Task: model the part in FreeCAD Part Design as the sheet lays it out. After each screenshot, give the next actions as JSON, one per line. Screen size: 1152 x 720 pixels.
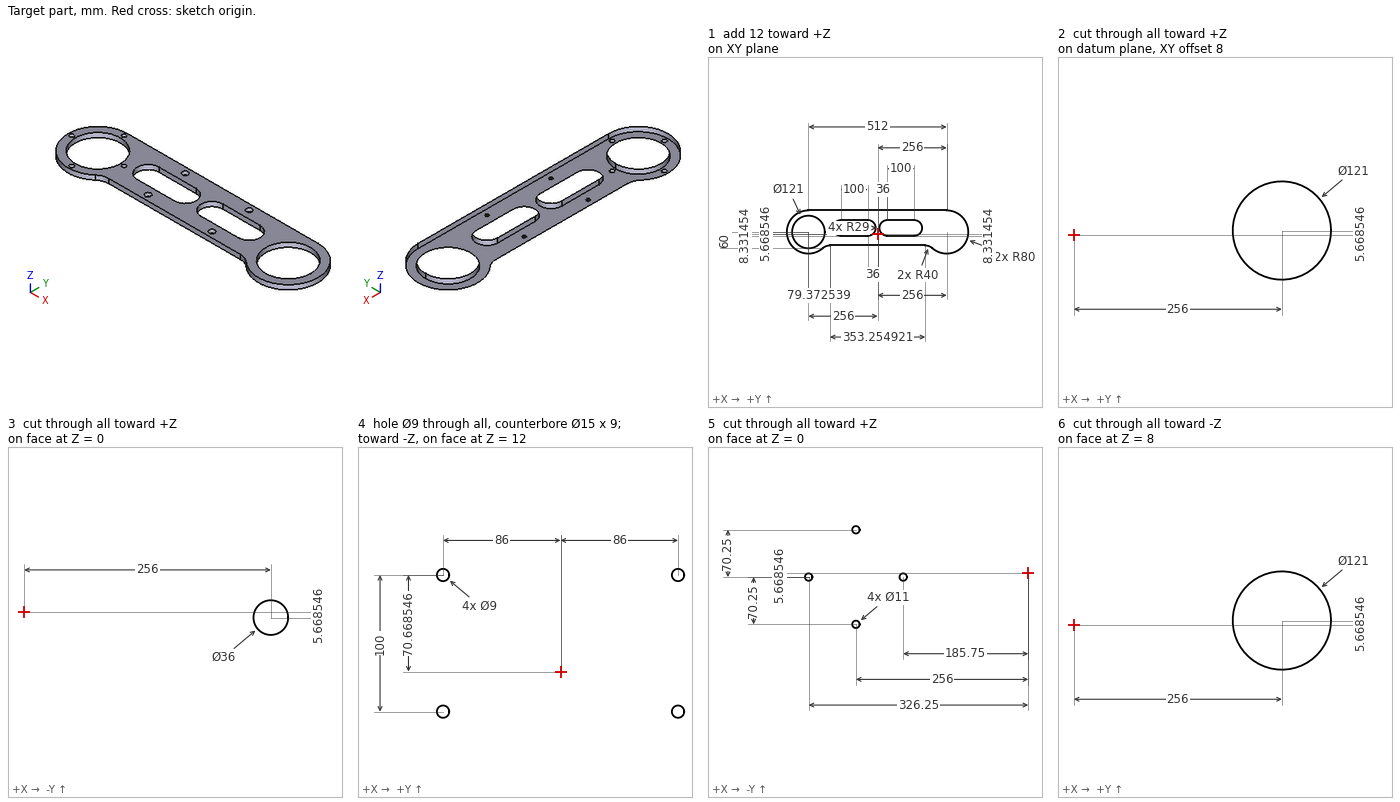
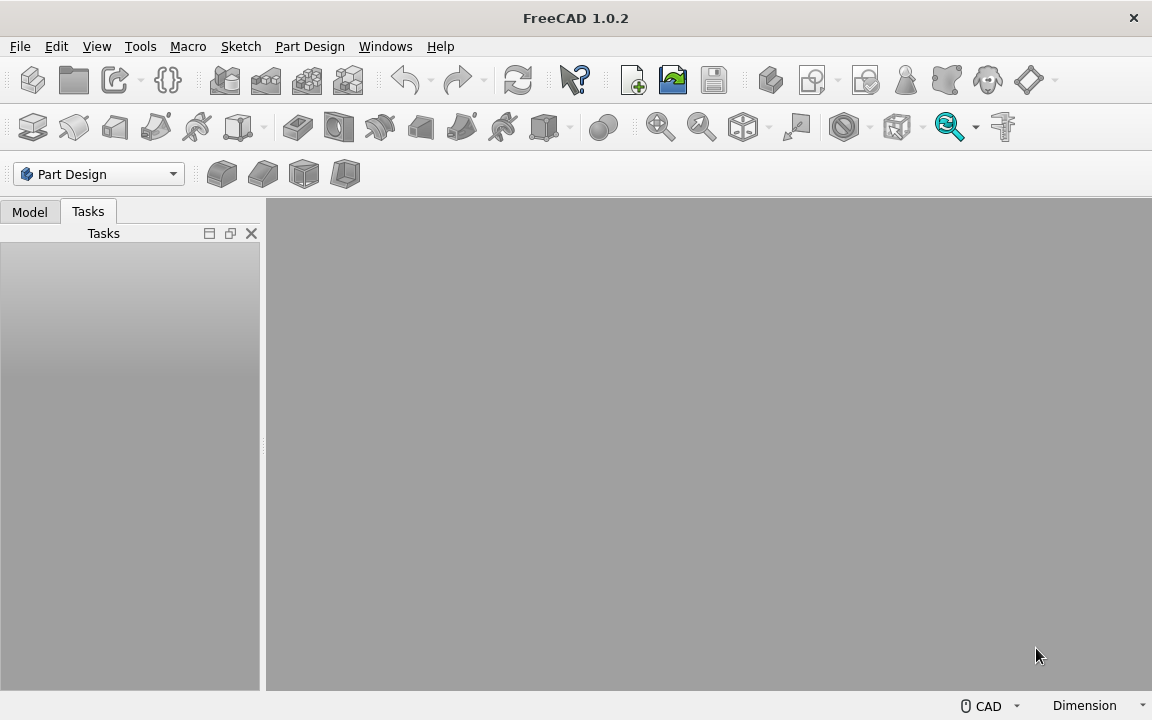
{"action": "left_click", "coordinate": [632, 80]}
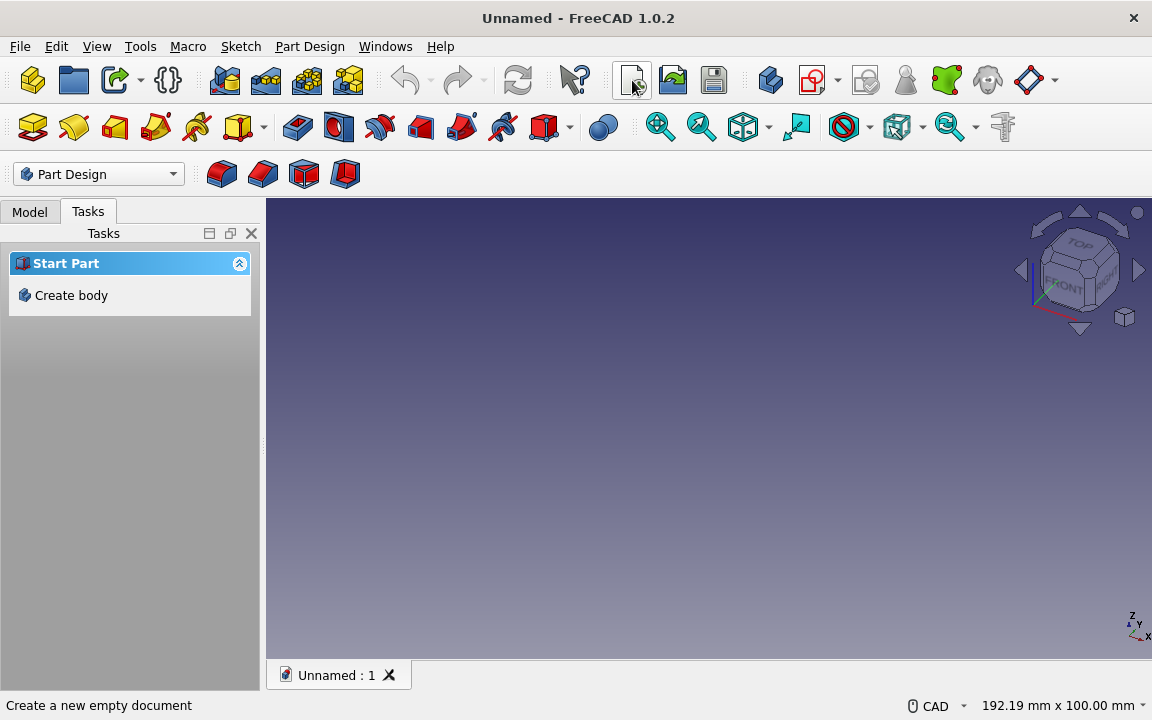
{"action": "left_click", "coordinate": [812, 80]}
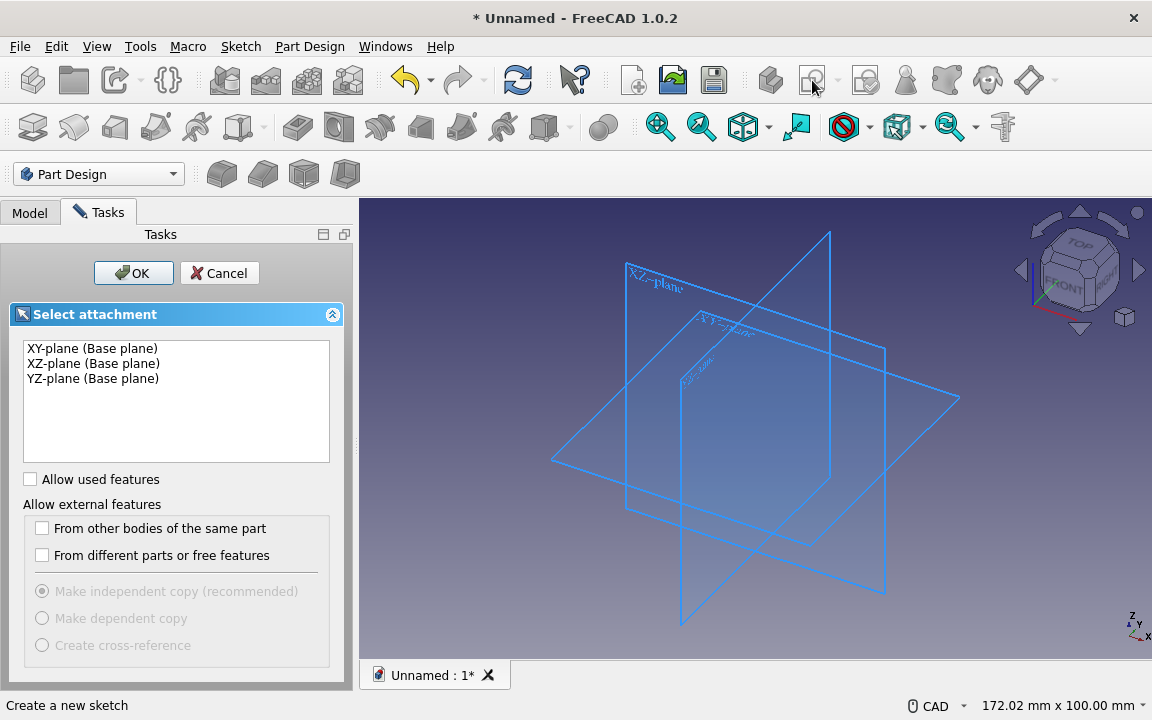
{"action": "left_click", "coordinate": [84, 348]}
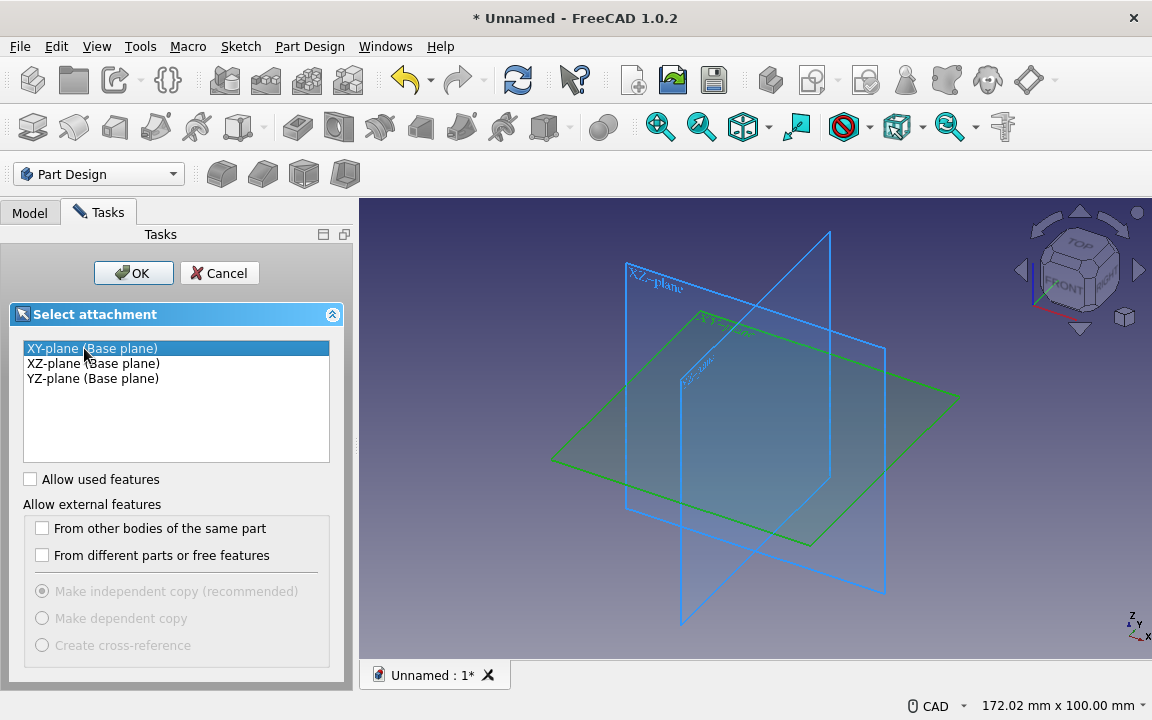
{"action": "left_click", "coordinate": [134, 273]}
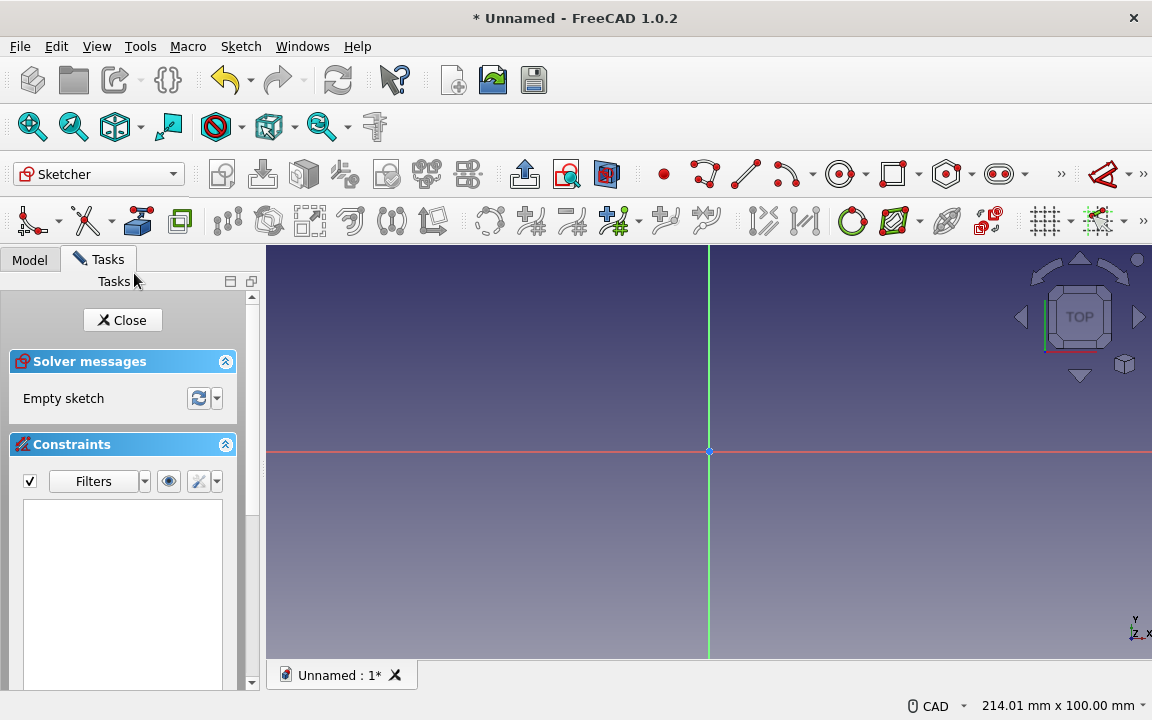
{"action": "scroll", "coordinate": [627, 465], "scroll_direction": "down", "scroll_amount": 9}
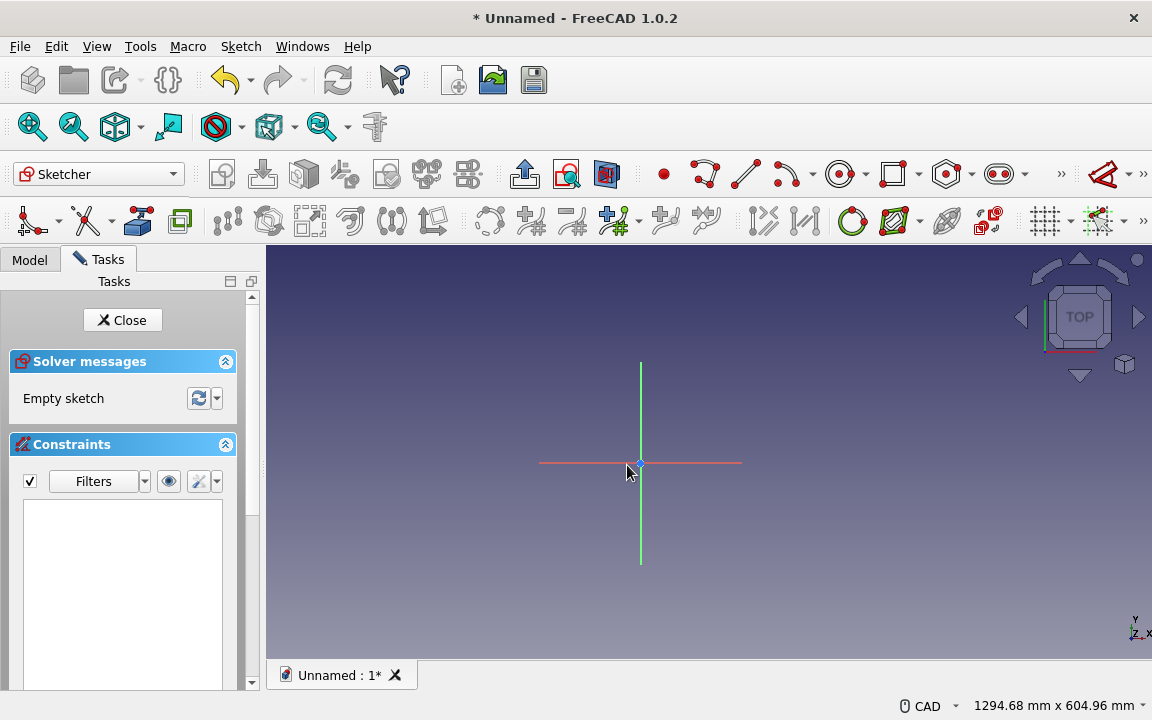
{"action": "left_click", "coordinate": [746, 174]}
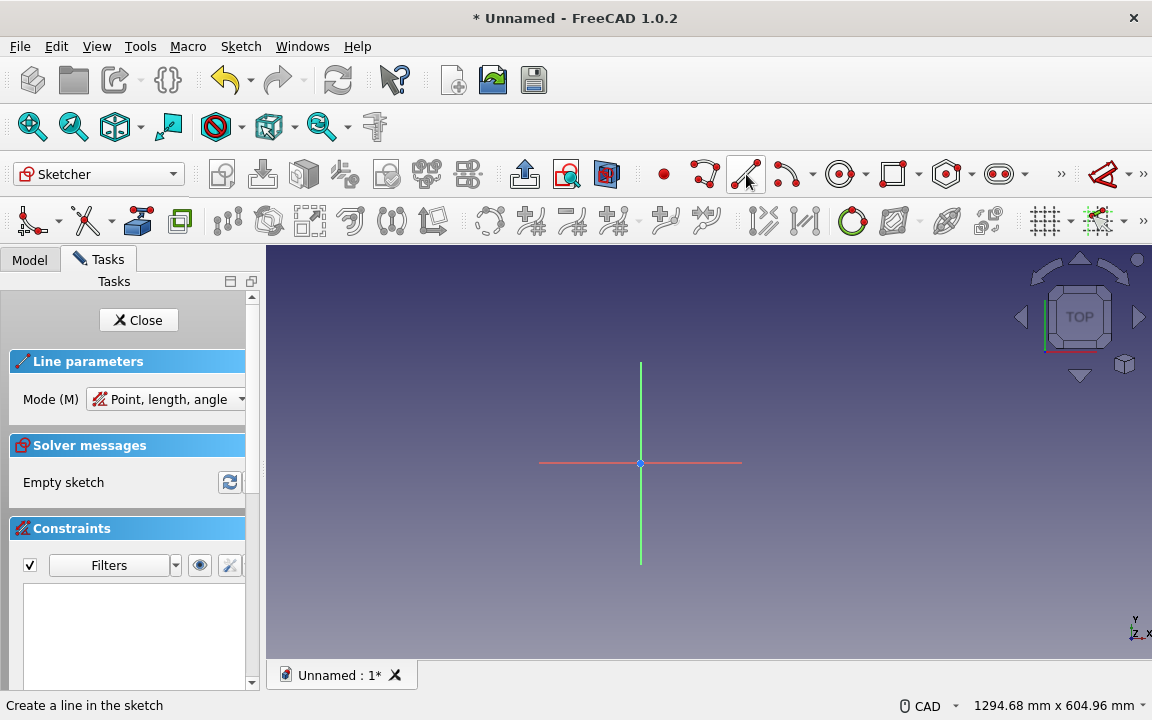
{"action": "left_click", "coordinate": [816, 405]}
{"action": "left_click", "coordinate": [466, 405]}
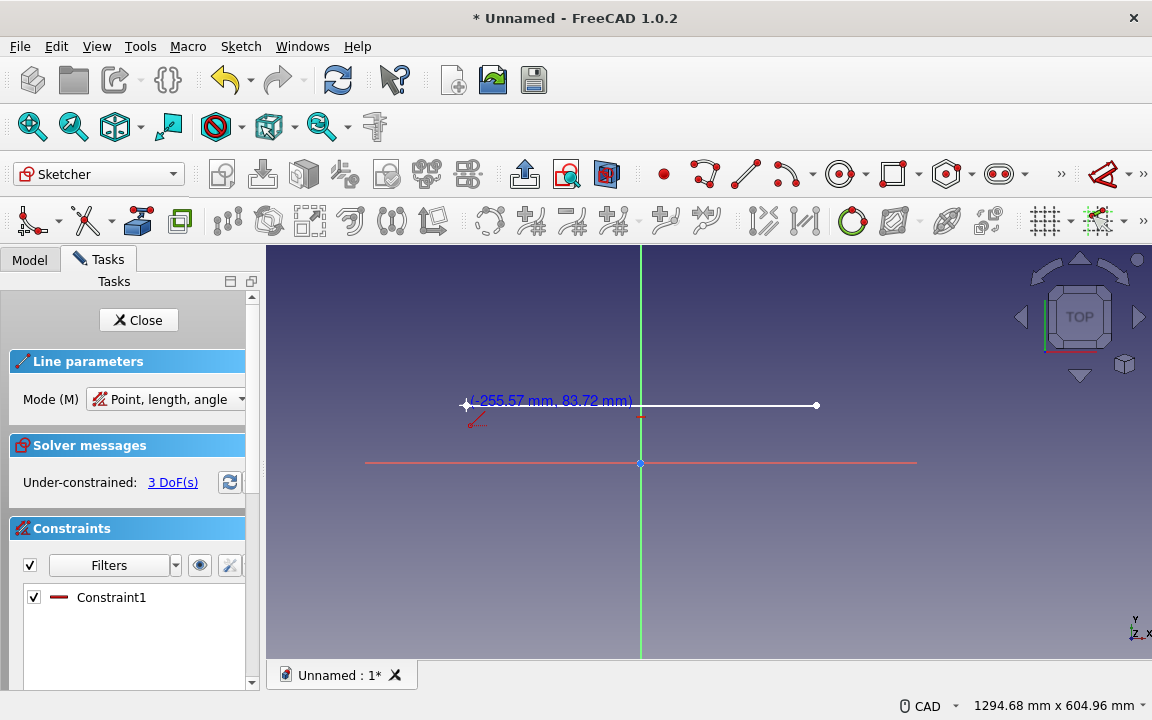
{"action": "left_click", "coordinate": [520, 494]}
{"action": "left_click", "coordinate": [762, 494]}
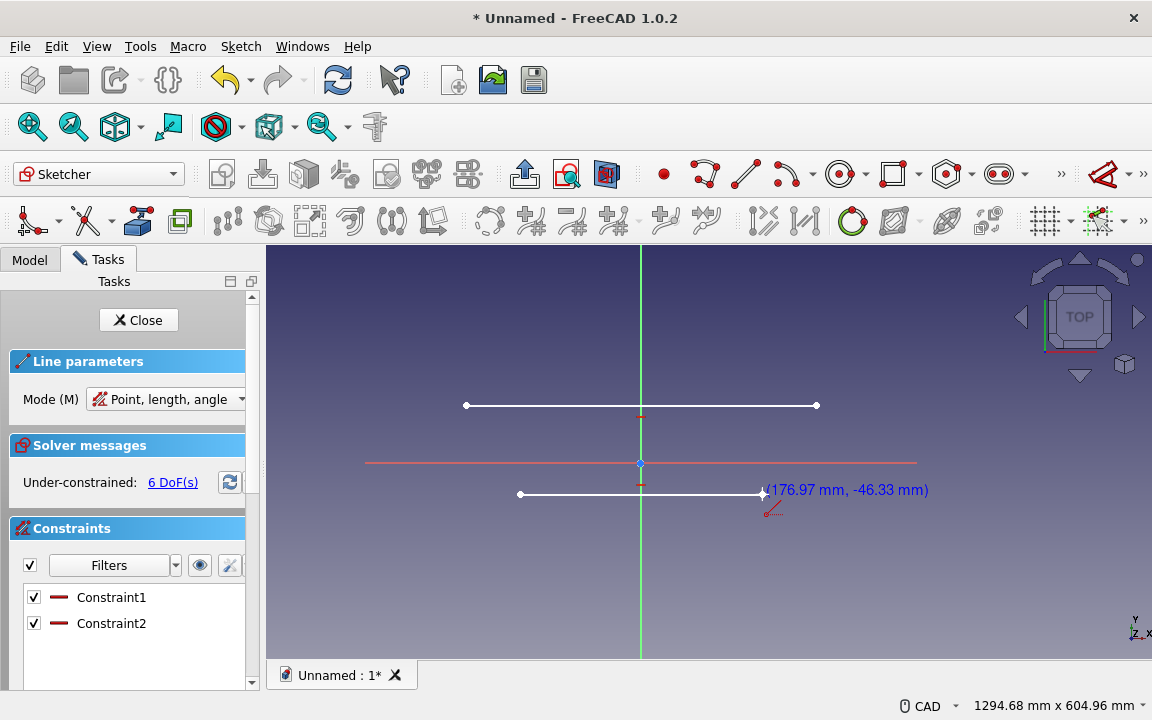
{"action": "left_click", "coordinate": [812, 174]}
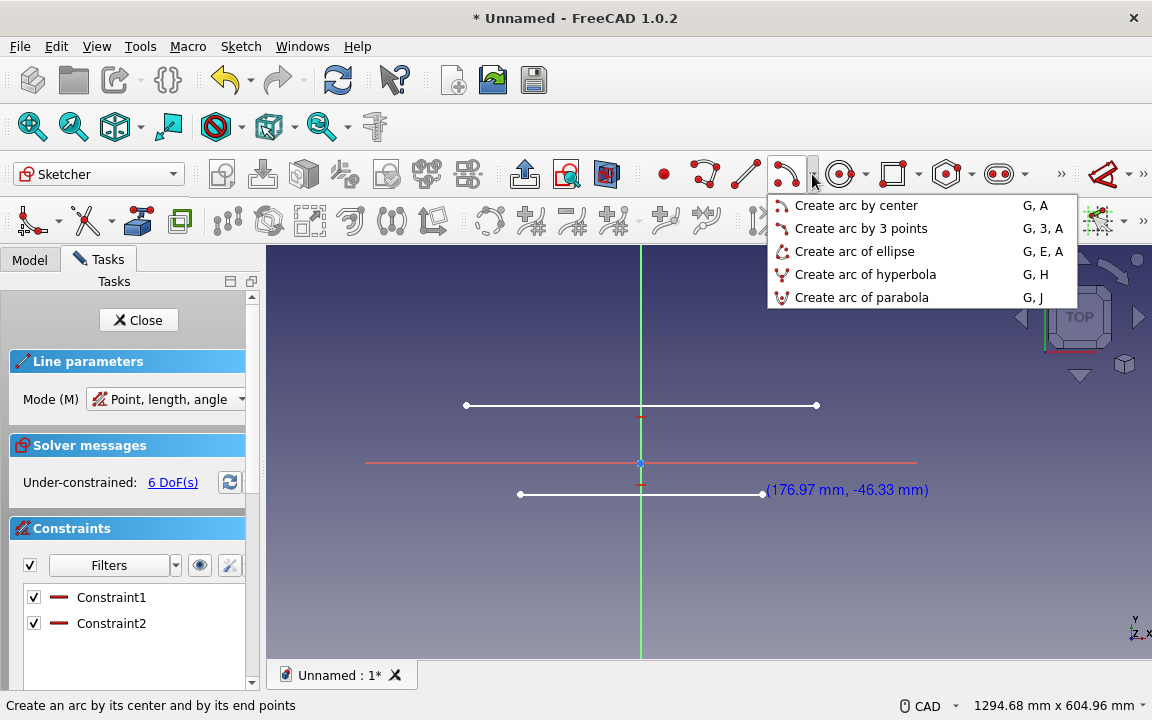
{"action": "left_click", "coordinate": [922, 228]}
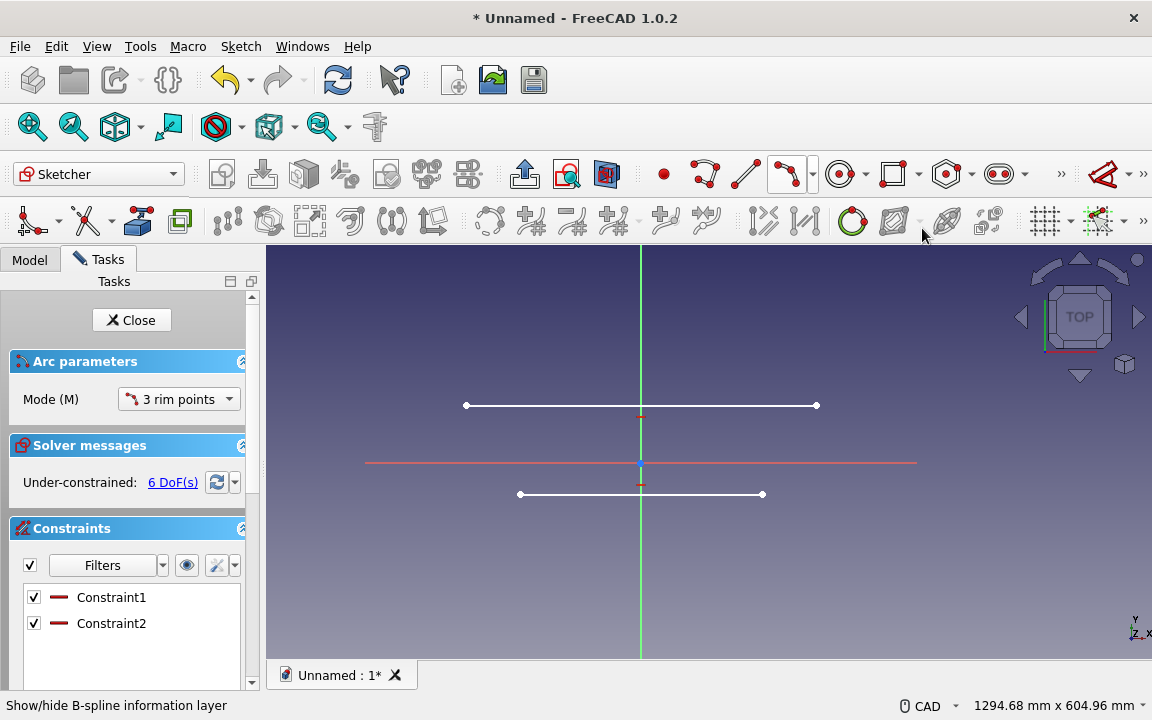
{"action": "left_click", "coordinate": [466, 406]}
{"action": "left_click", "coordinate": [502, 500]}
{"action": "left_click", "coordinate": [414, 479]}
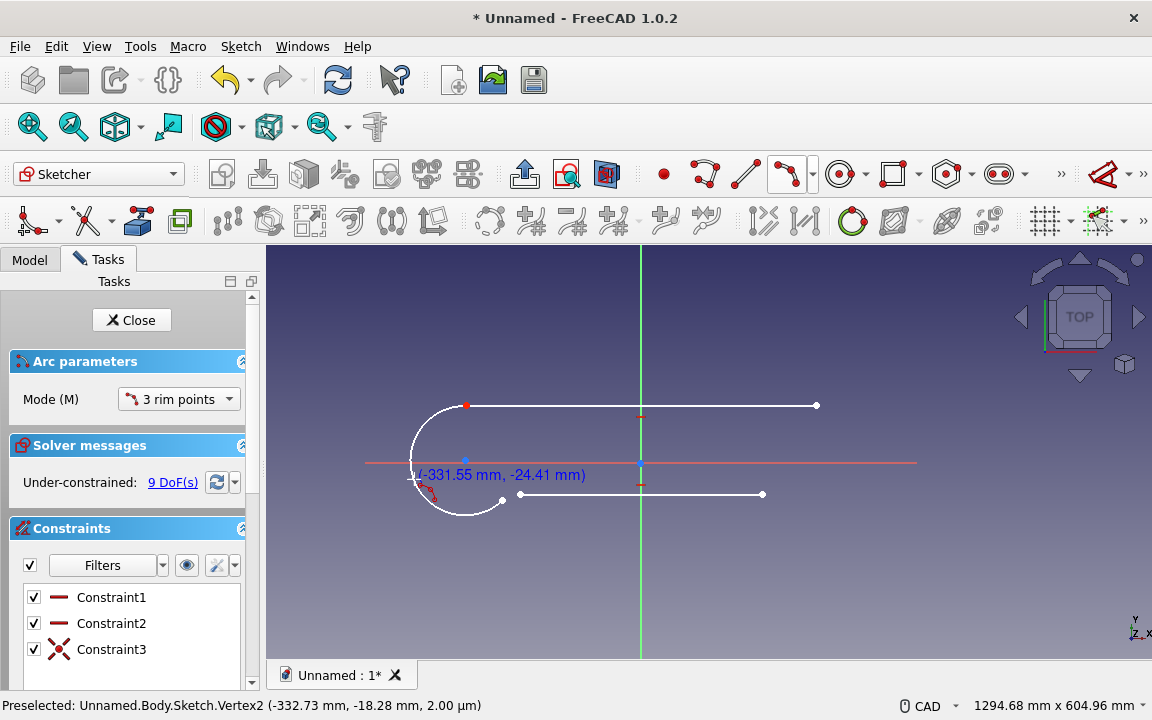
{"action": "left_click", "coordinate": [502, 501]}
{"action": "left_click", "coordinate": [520, 495]}